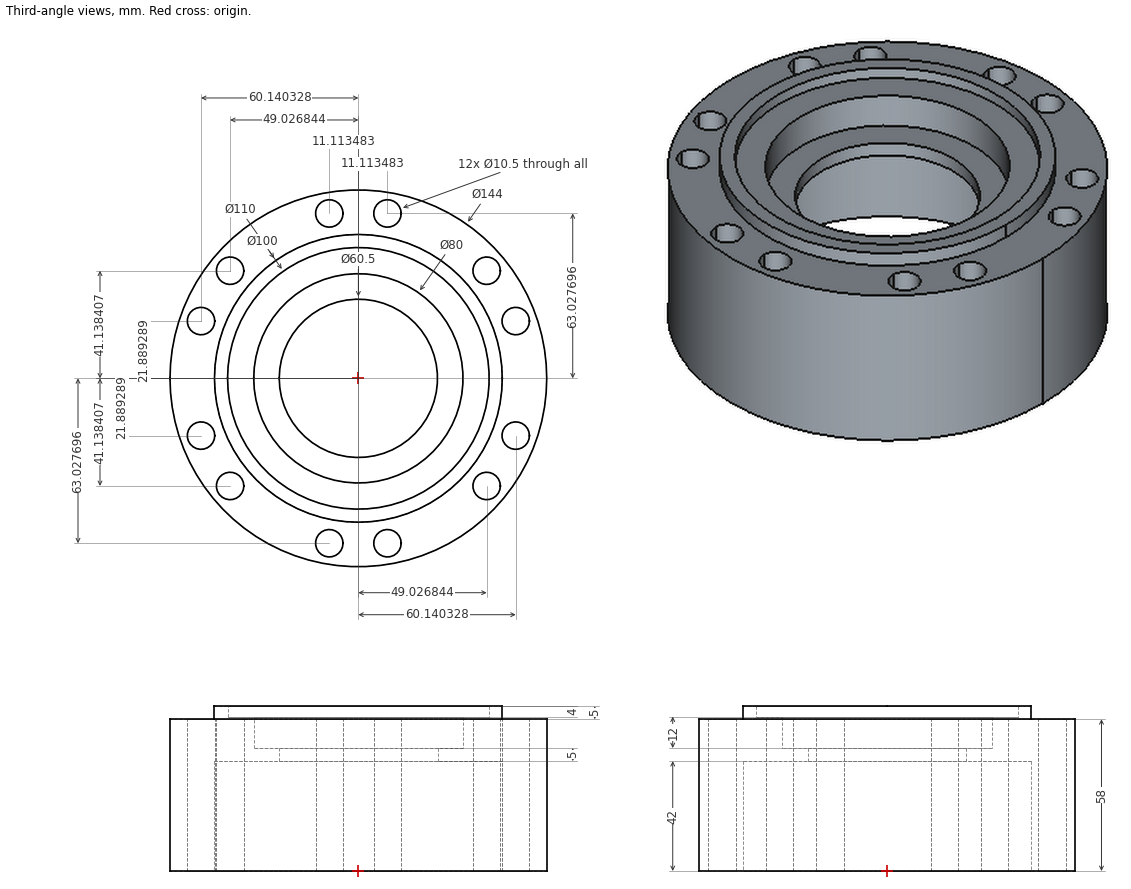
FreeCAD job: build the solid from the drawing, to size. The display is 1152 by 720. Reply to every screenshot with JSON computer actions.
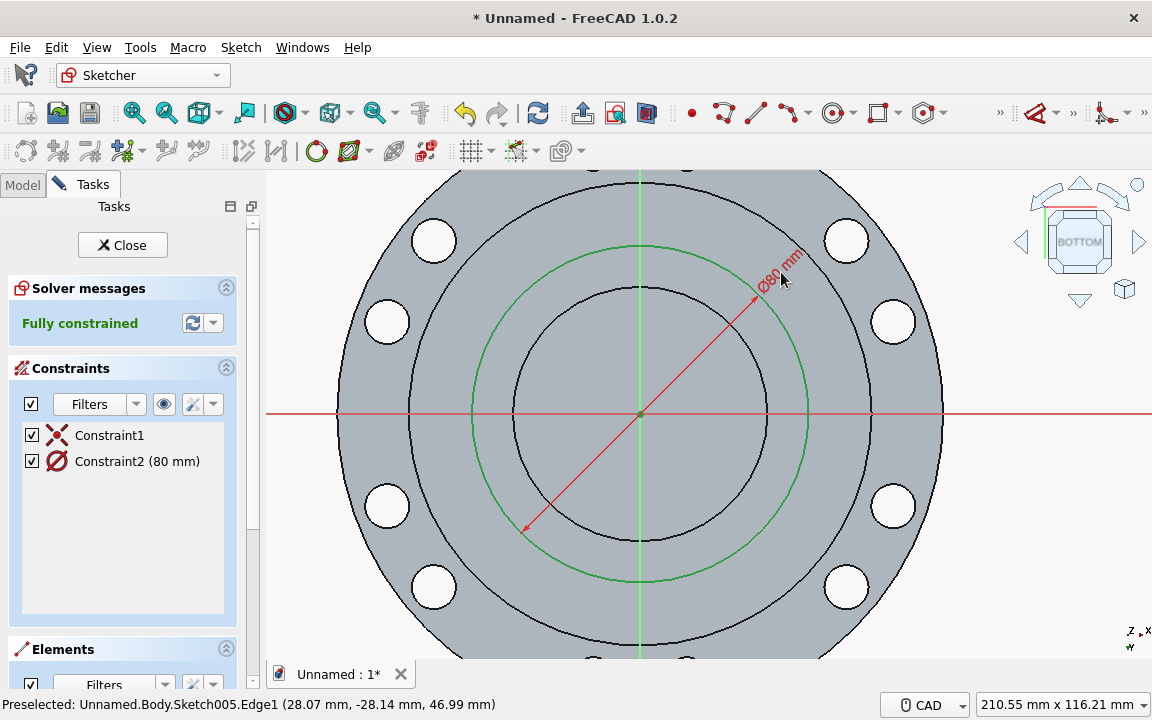
{"action": "left_click", "coordinate": [123, 245]}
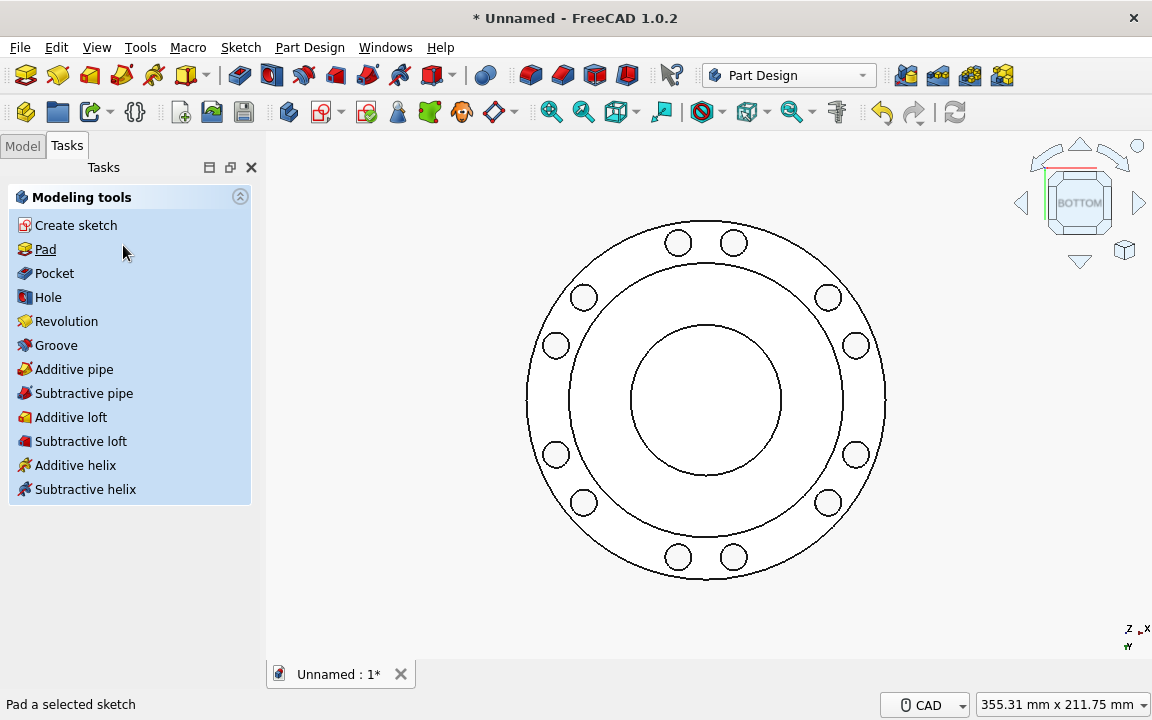
{"action": "left_click", "coordinate": [240, 76]}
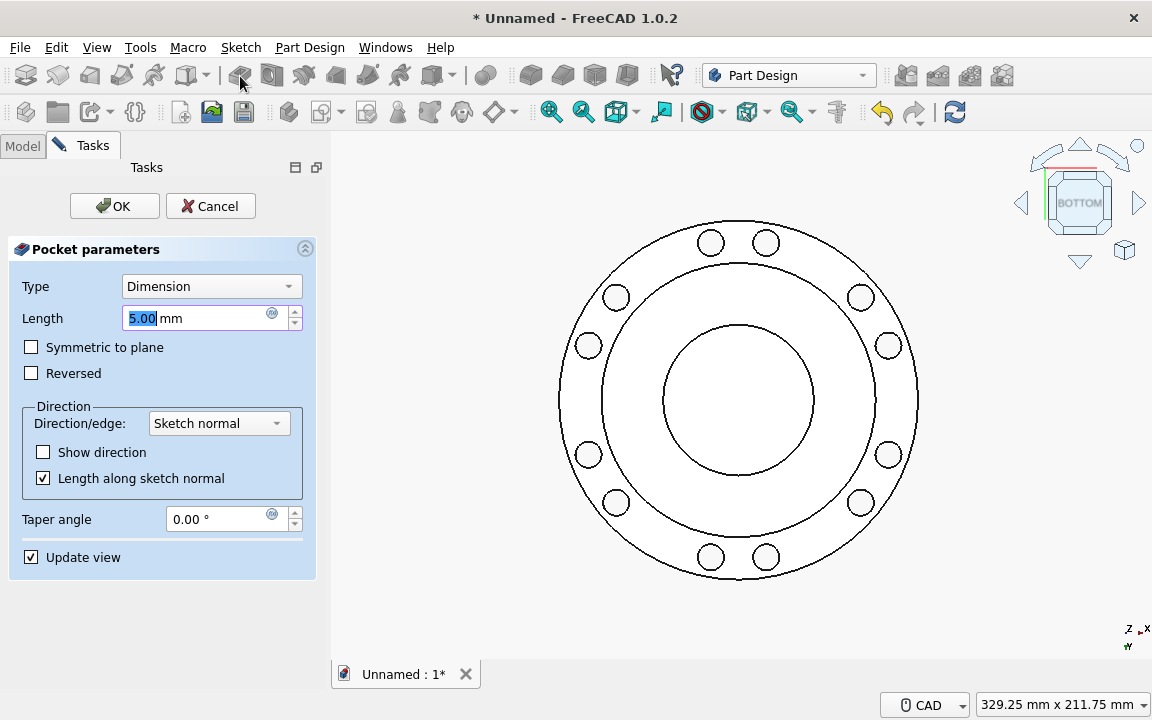
{"action": "type", "text": "12"}
{"action": "key", "text": "Tab"}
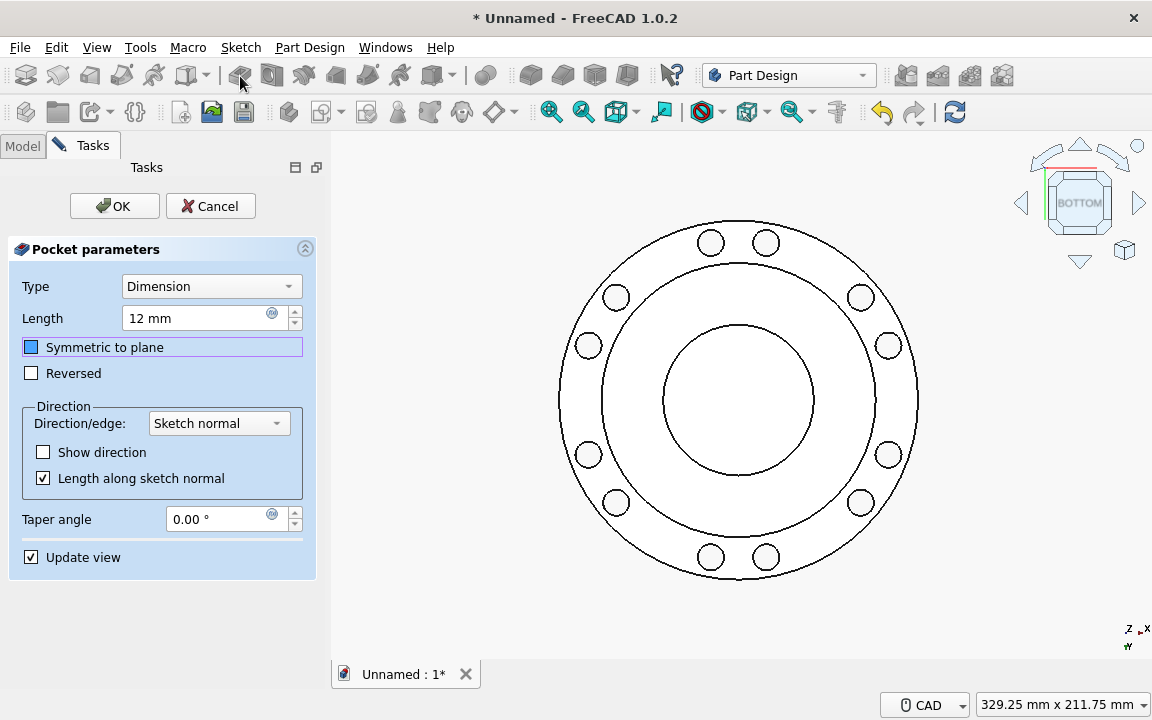
{"action": "left_click", "coordinate": [115, 206]}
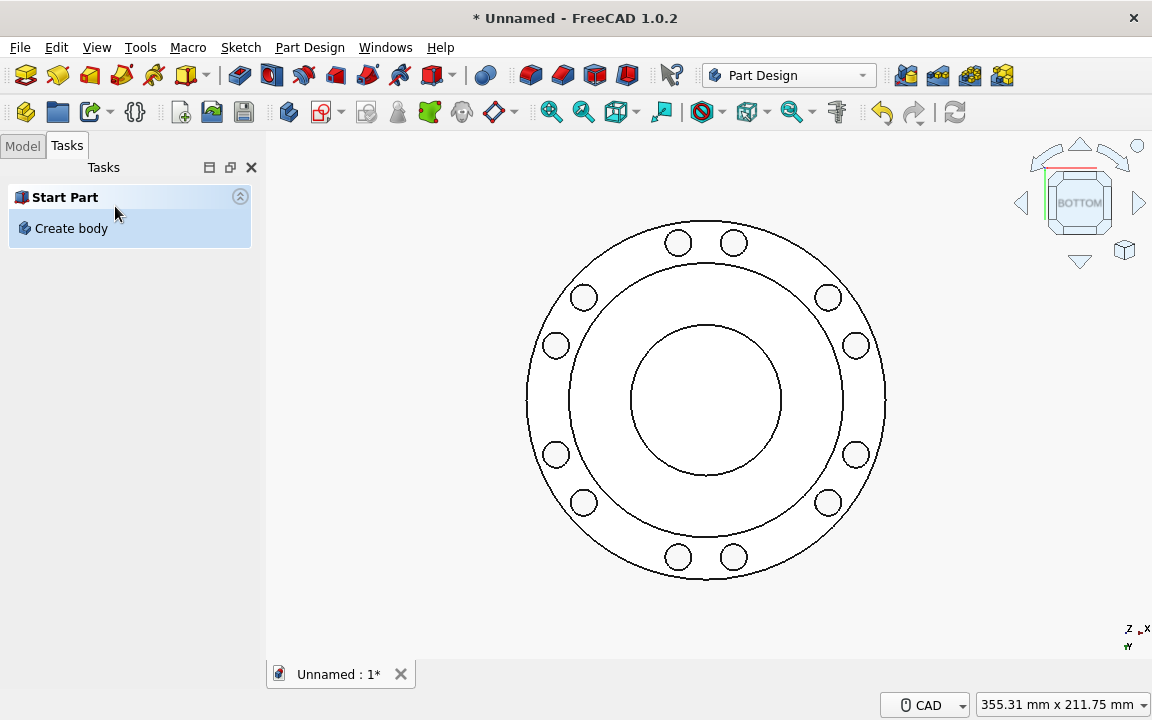
{"action": "left_click", "coordinate": [706, 399]}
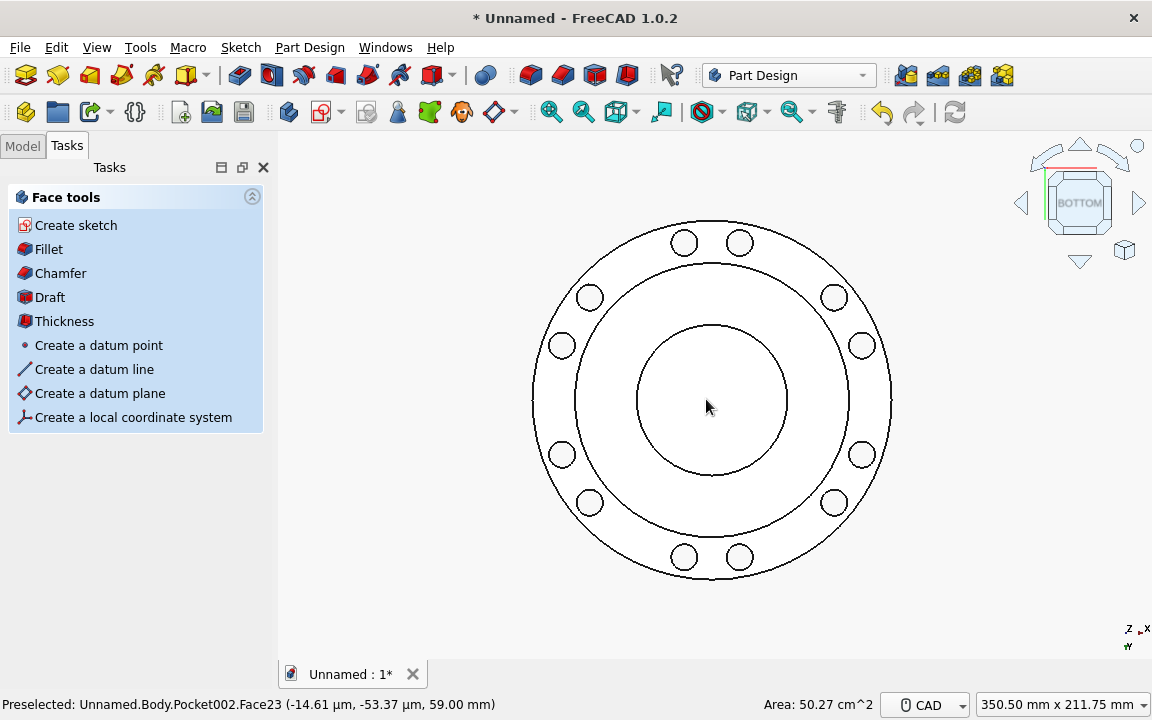
{"action": "left_click", "coordinate": [322, 112]}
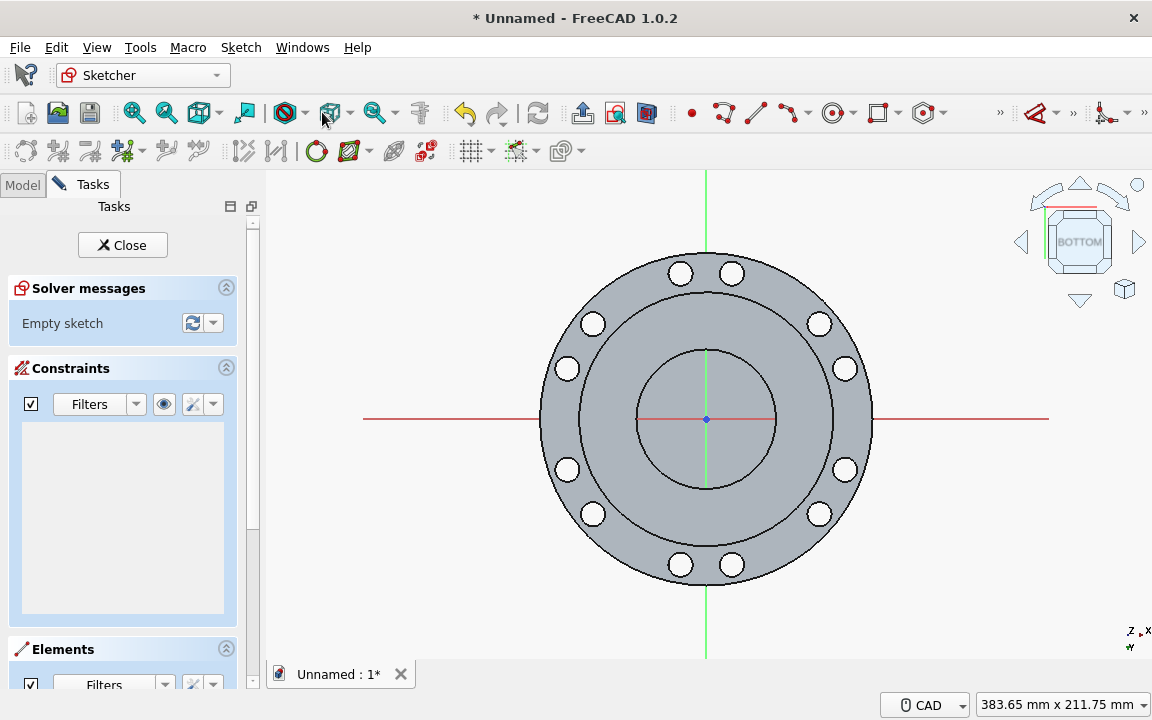
{"action": "key", "text": "g c"}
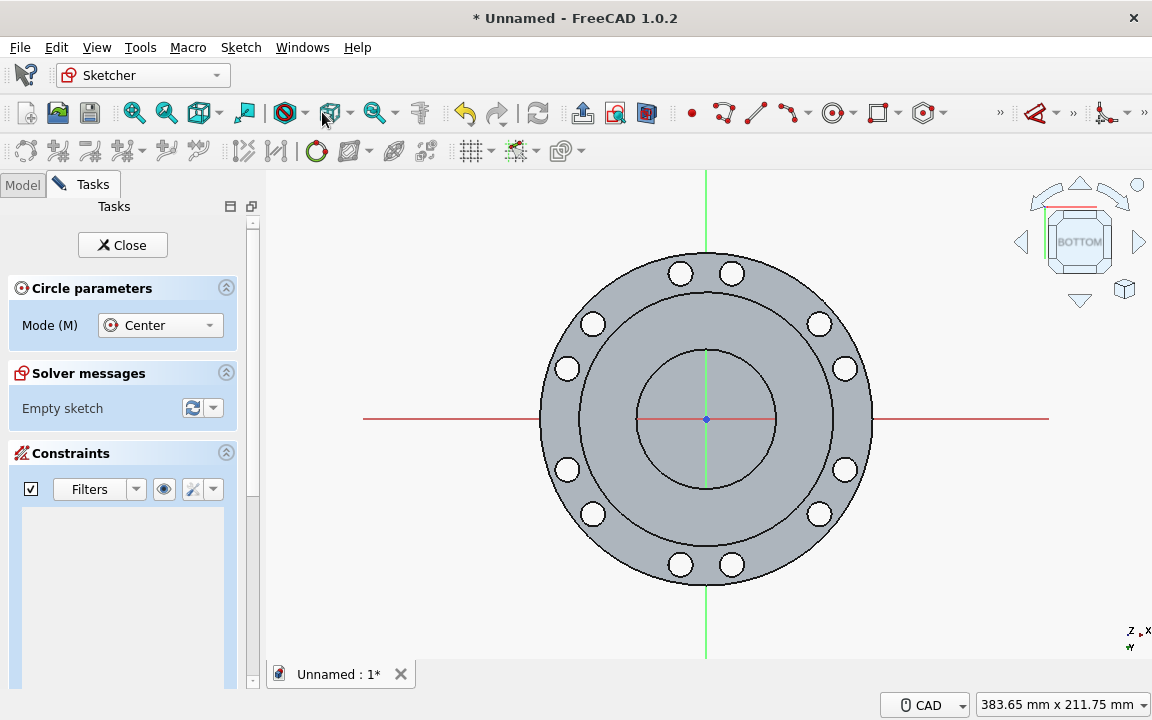
{"action": "left_click", "coordinate": [706, 419]}
{"action": "left_click", "coordinate": [788, 338]}
{"action": "key", "text": "Escape"}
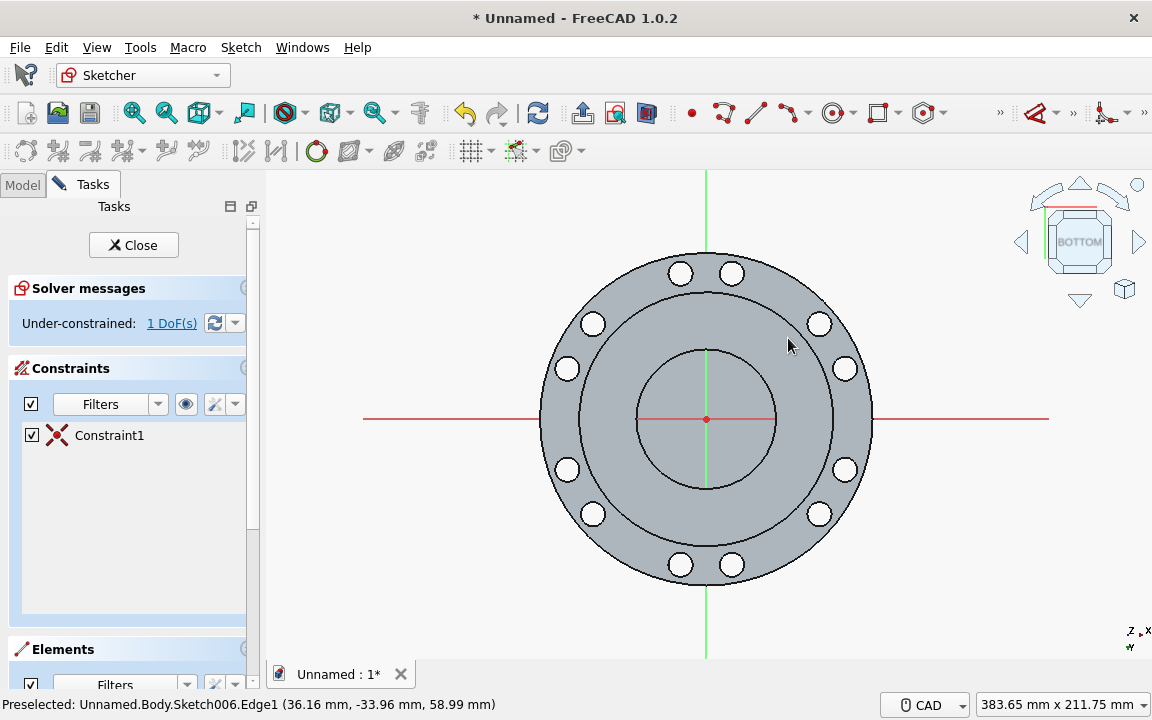
{"action": "key", "text": "d"}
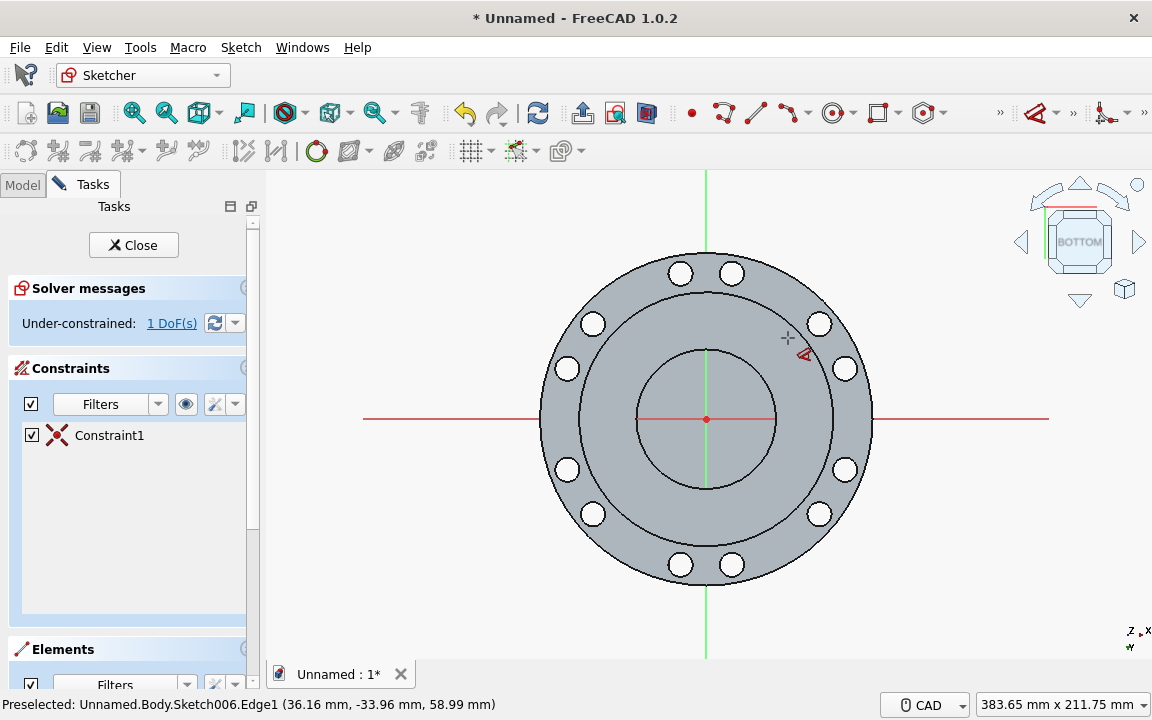
{"action": "left_click", "coordinate": [787, 338]}
{"action": "left_click", "coordinate": [810, 315]}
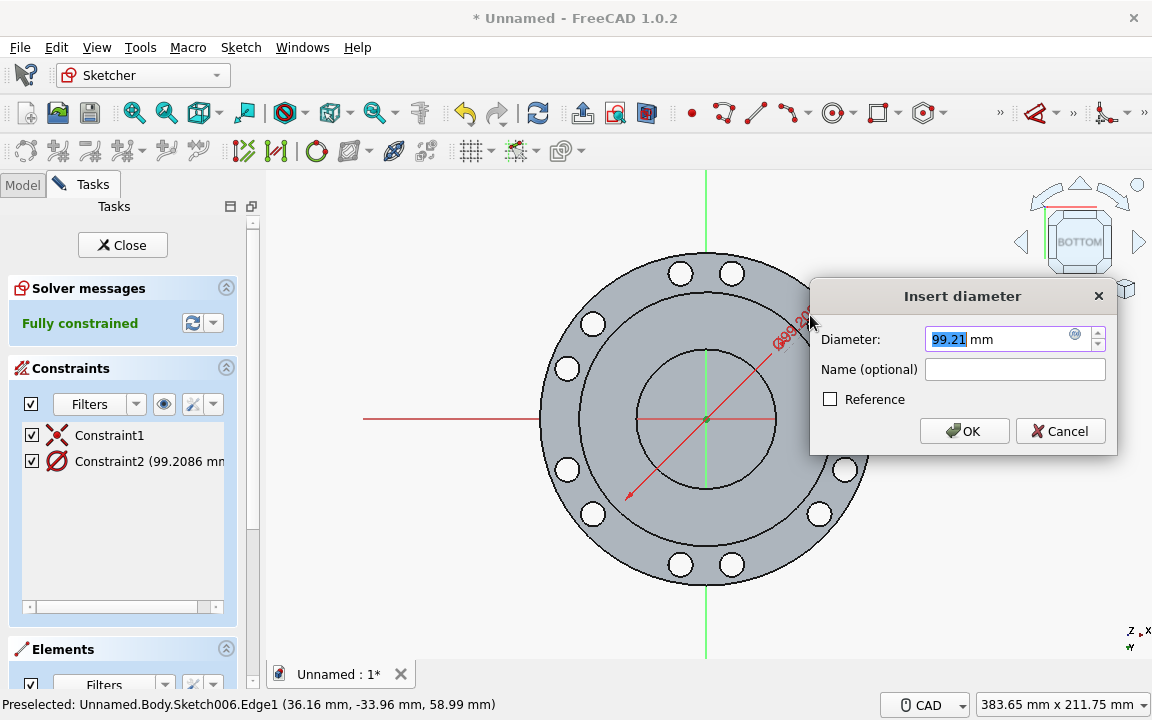
{"action": "type", "text": "100"}
{"action": "key", "text": "Return"}
{"action": "key", "text": "Escape"}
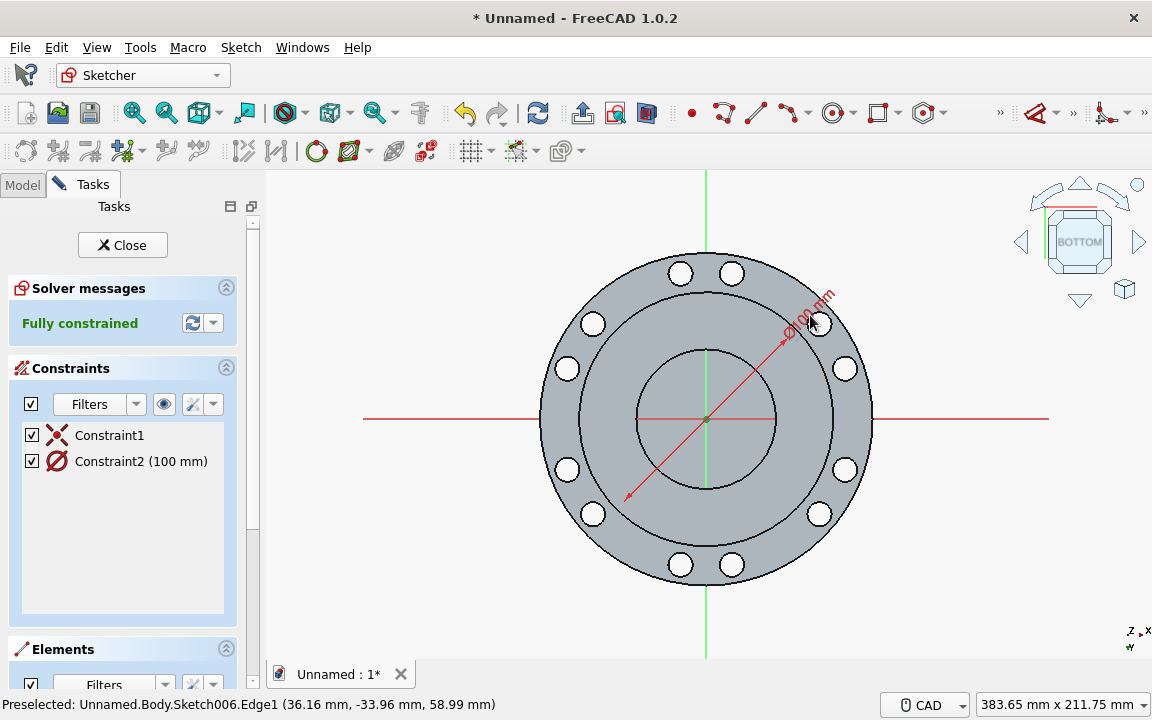
{"action": "left_click", "coordinate": [123, 245]}